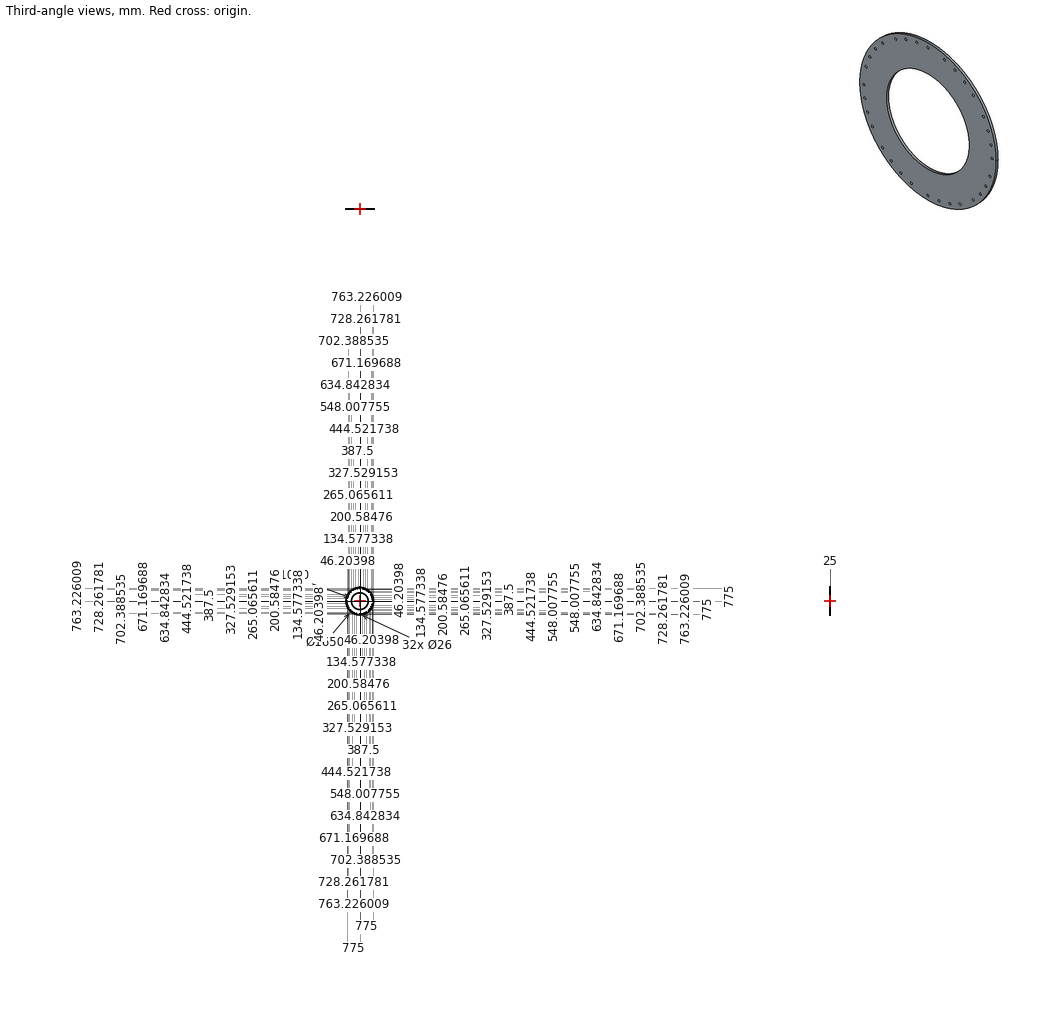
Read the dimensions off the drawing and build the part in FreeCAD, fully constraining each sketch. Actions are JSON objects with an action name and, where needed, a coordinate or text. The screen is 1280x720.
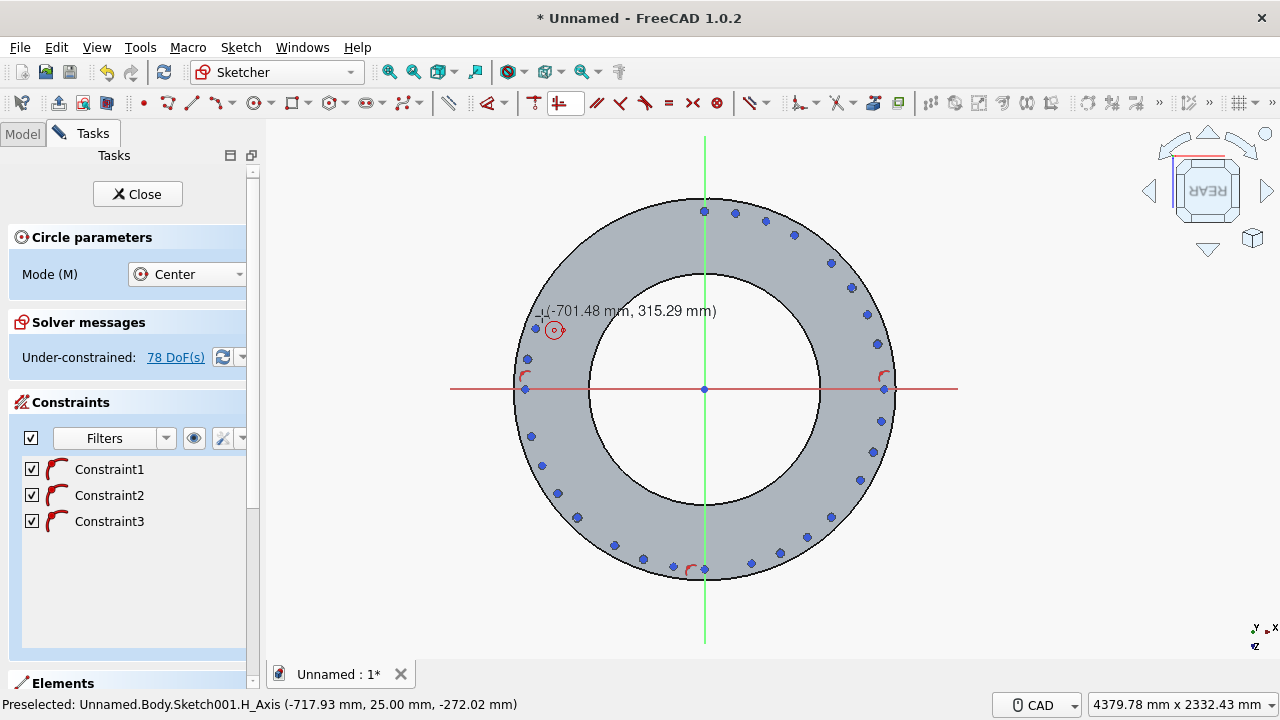
{"action": "left_click", "coordinate": [549, 300]}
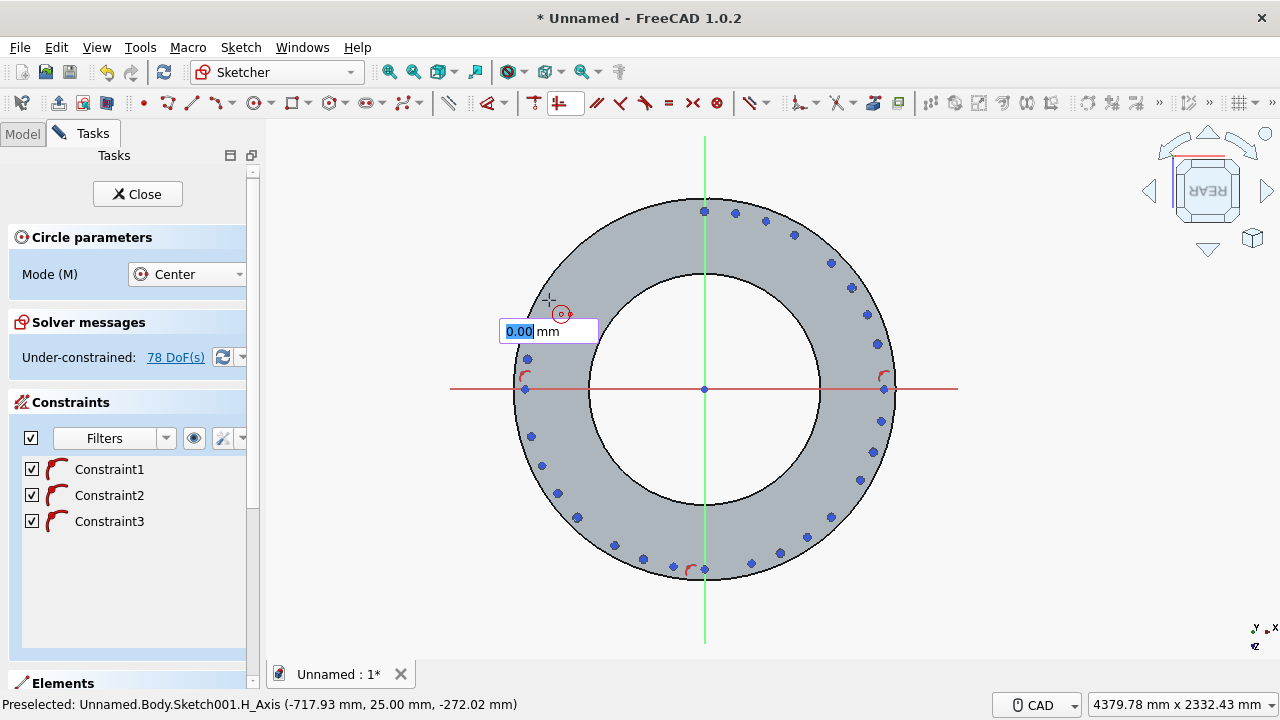
{"action": "scroll", "coordinate": [551, 298], "scroll_direction": "up", "scroll_amount": 9}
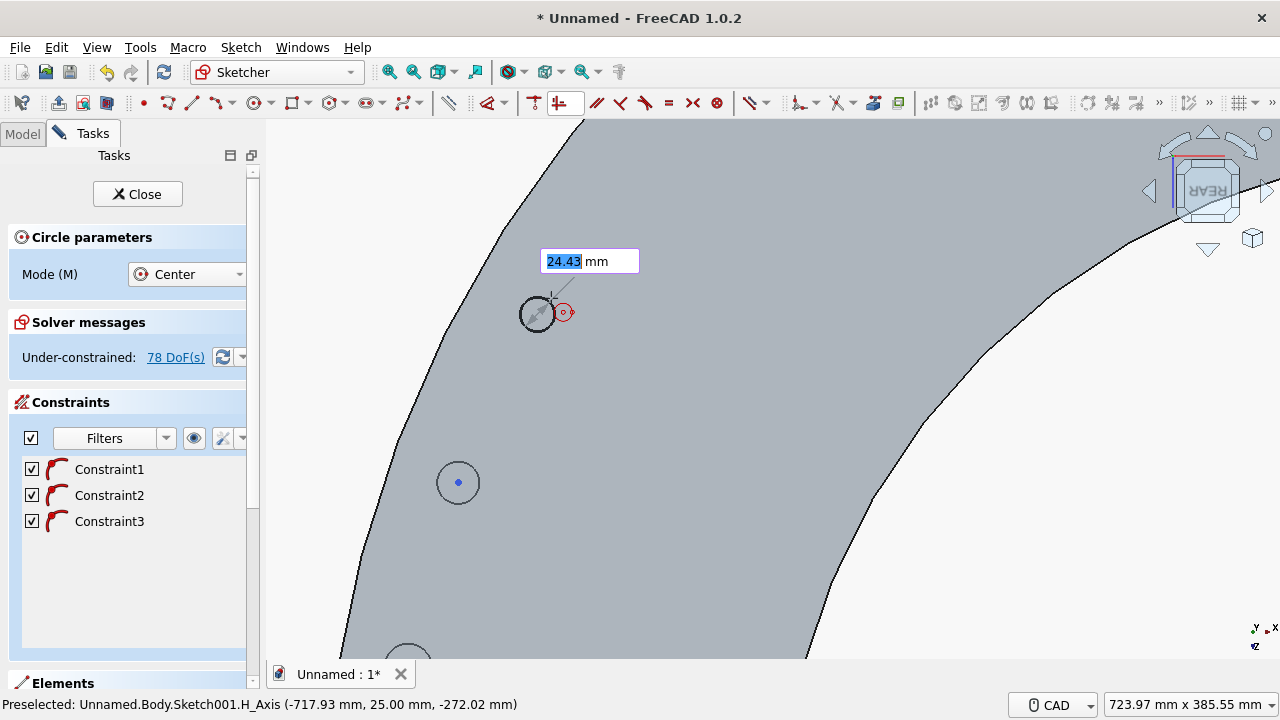
{"action": "left_click", "coordinate": [552, 294]}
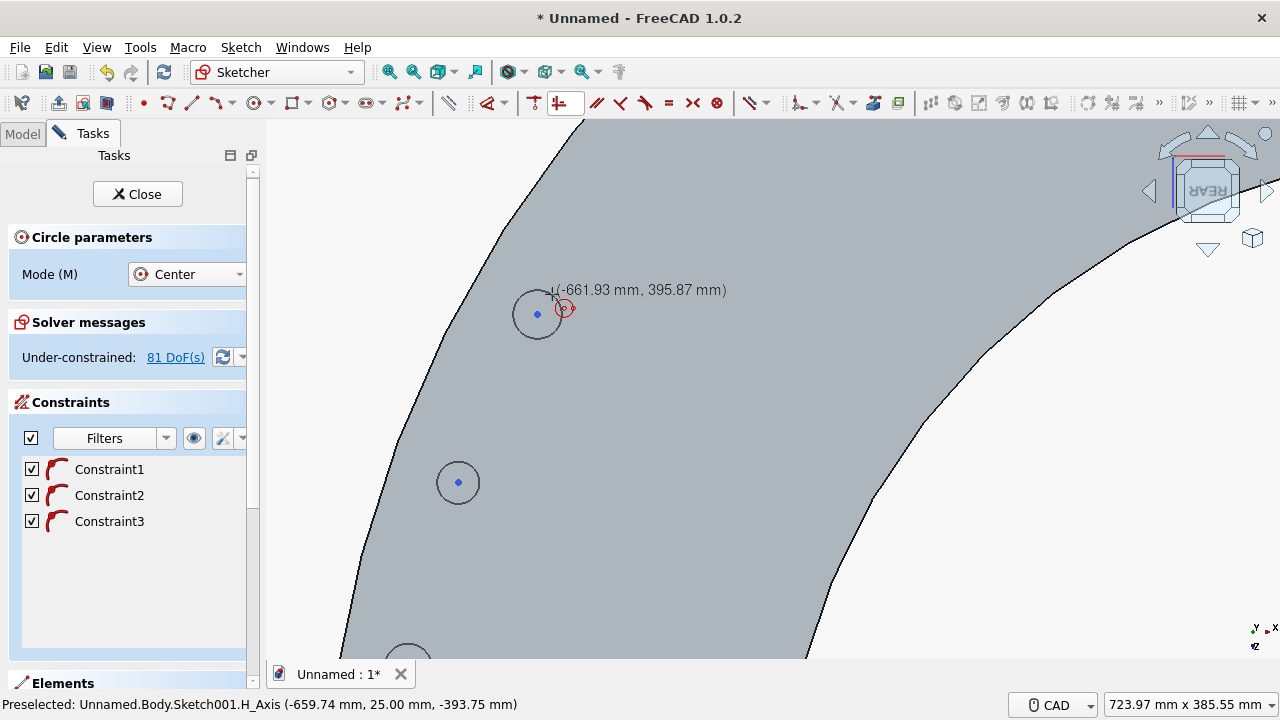
{"action": "scroll", "coordinate": [551, 298], "scroll_direction": "down", "scroll_amount": 9}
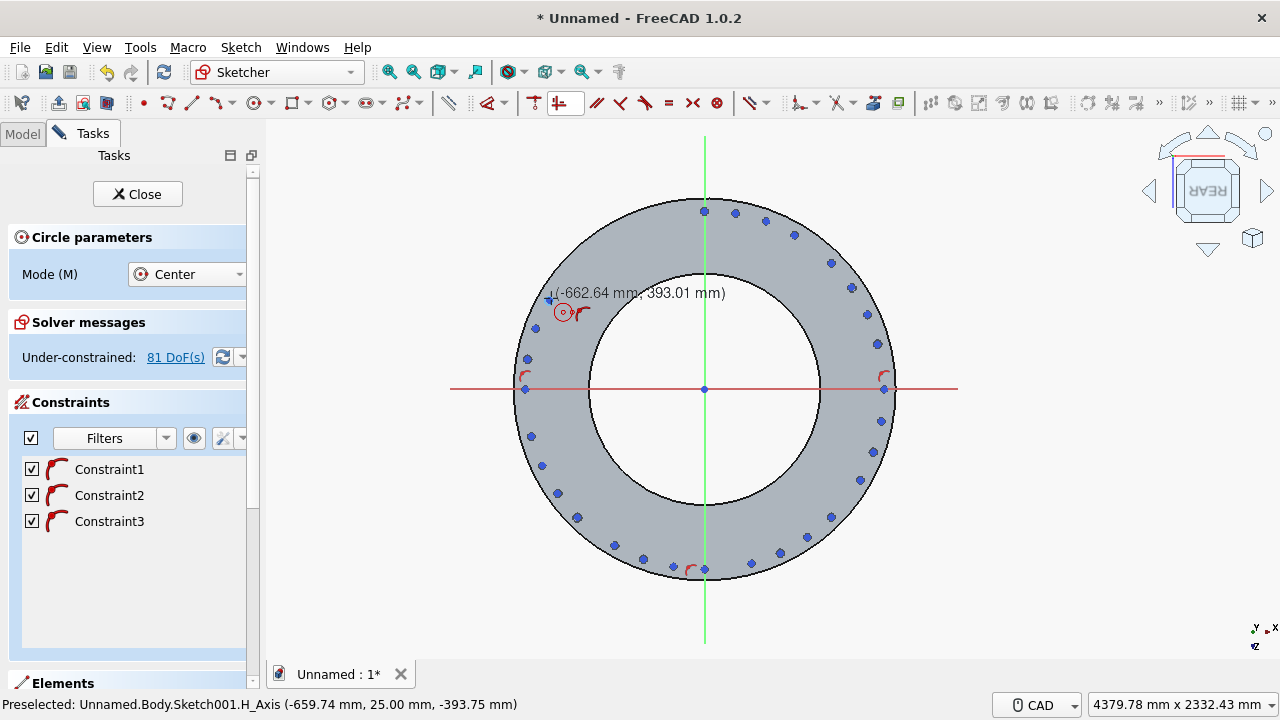
{"action": "scroll", "coordinate": [578, 263], "scroll_direction": "up", "scroll_amount": 11}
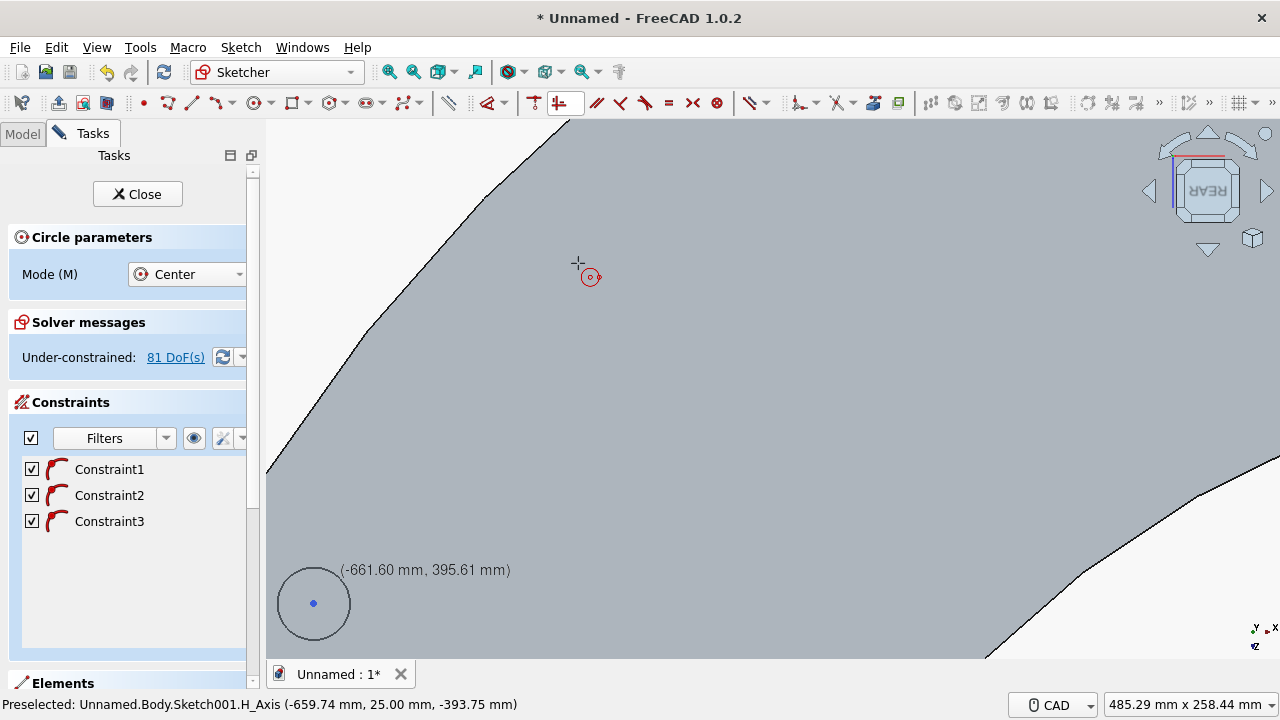
{"action": "scroll", "coordinate": [578, 263], "scroll_direction": "down", "scroll_amount": 11}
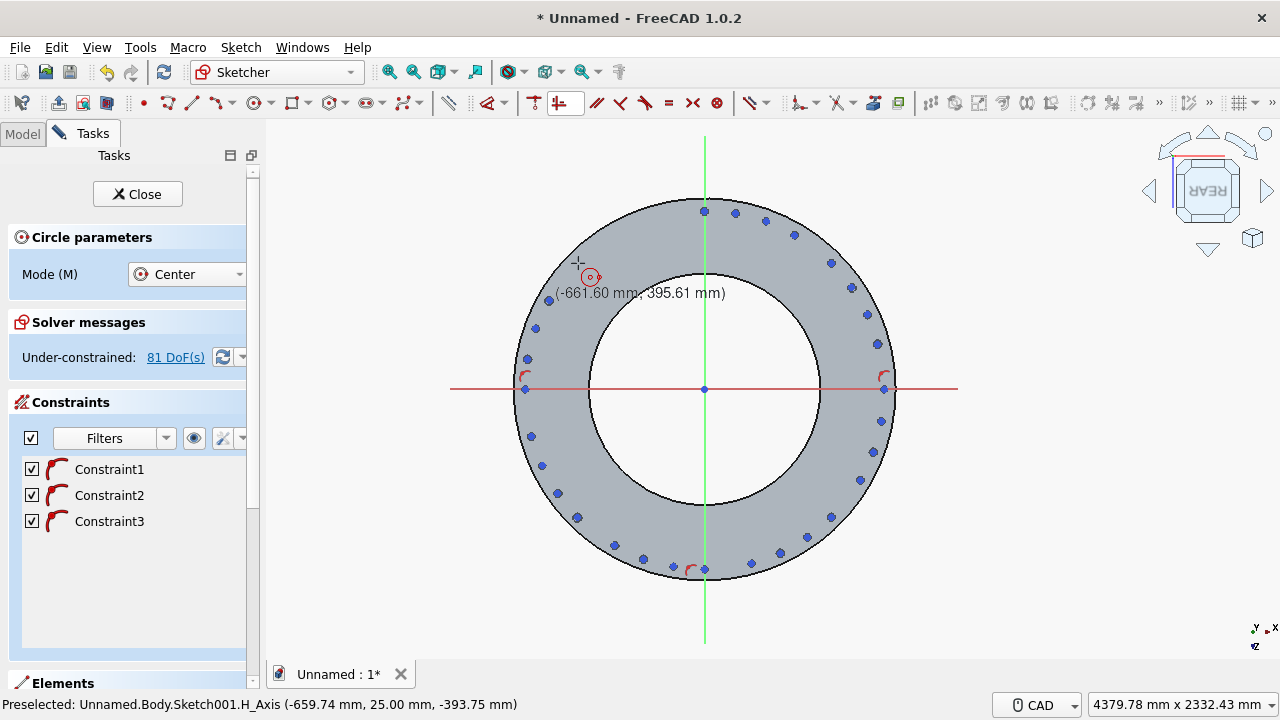
{"action": "left_click", "coordinate": [578, 263]}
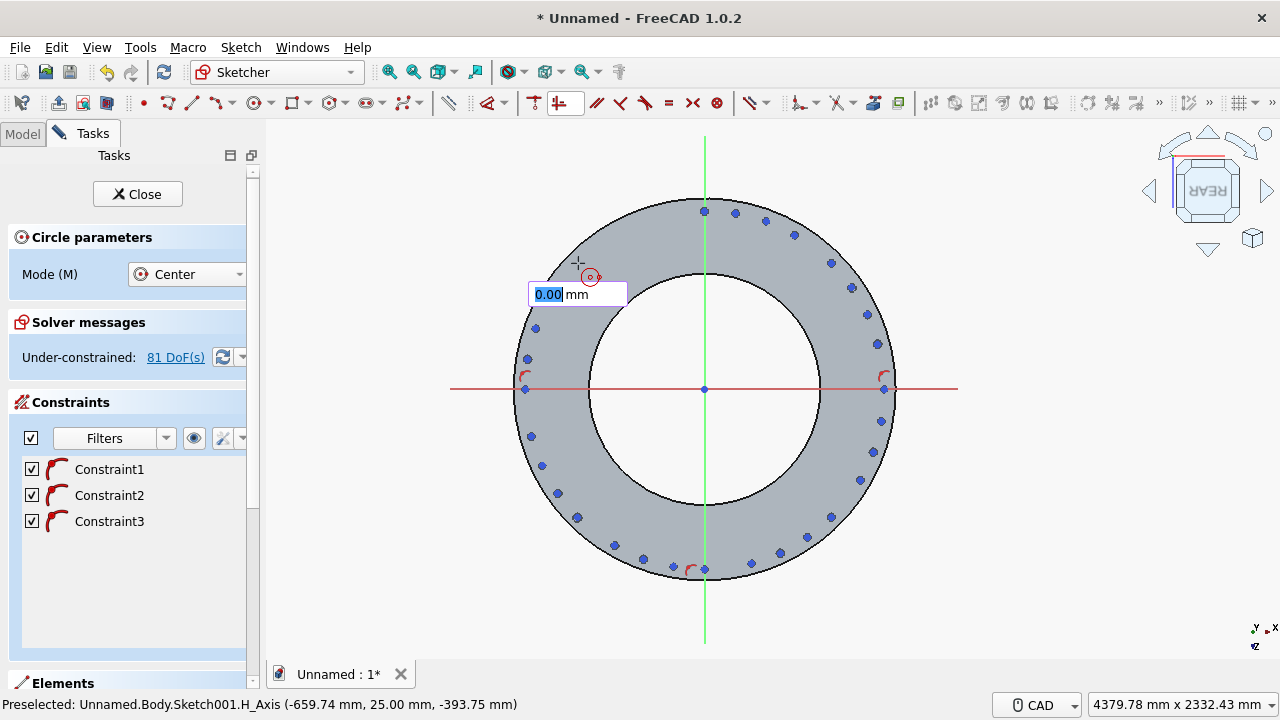
{"action": "scroll", "coordinate": [580, 260], "scroll_direction": "up", "scroll_amount": 9}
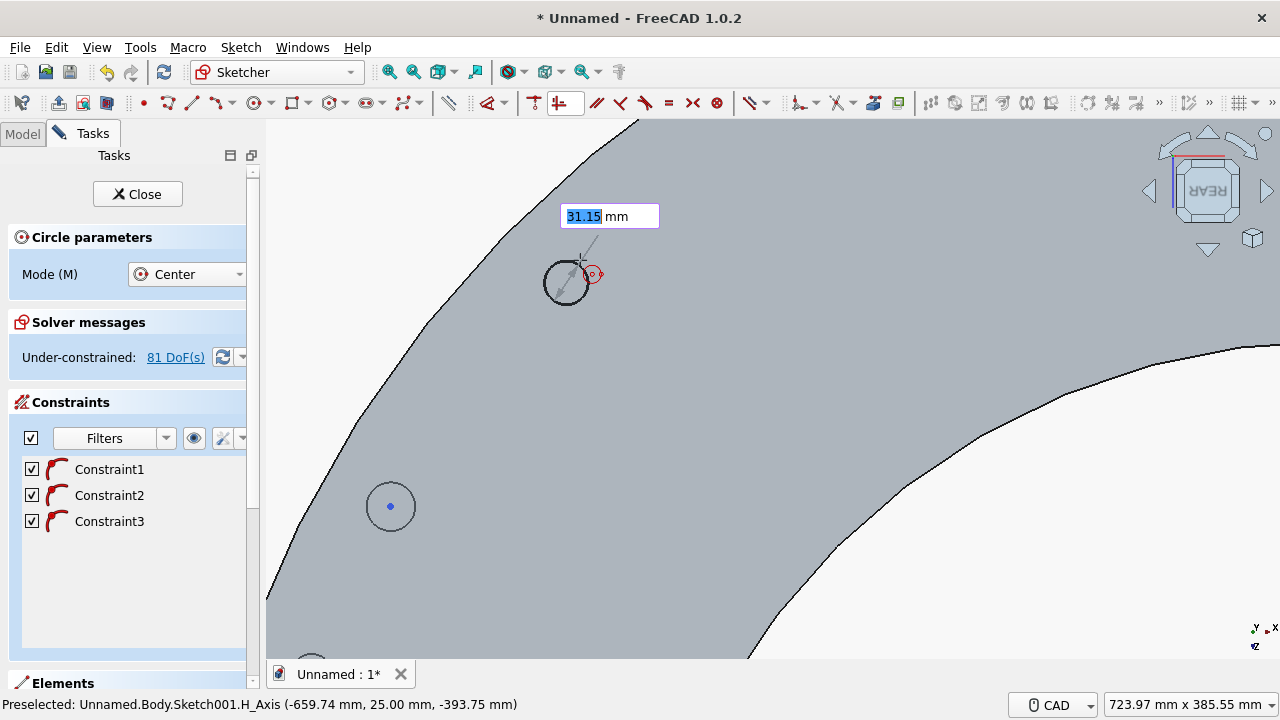
{"action": "left_click", "coordinate": [578, 261]}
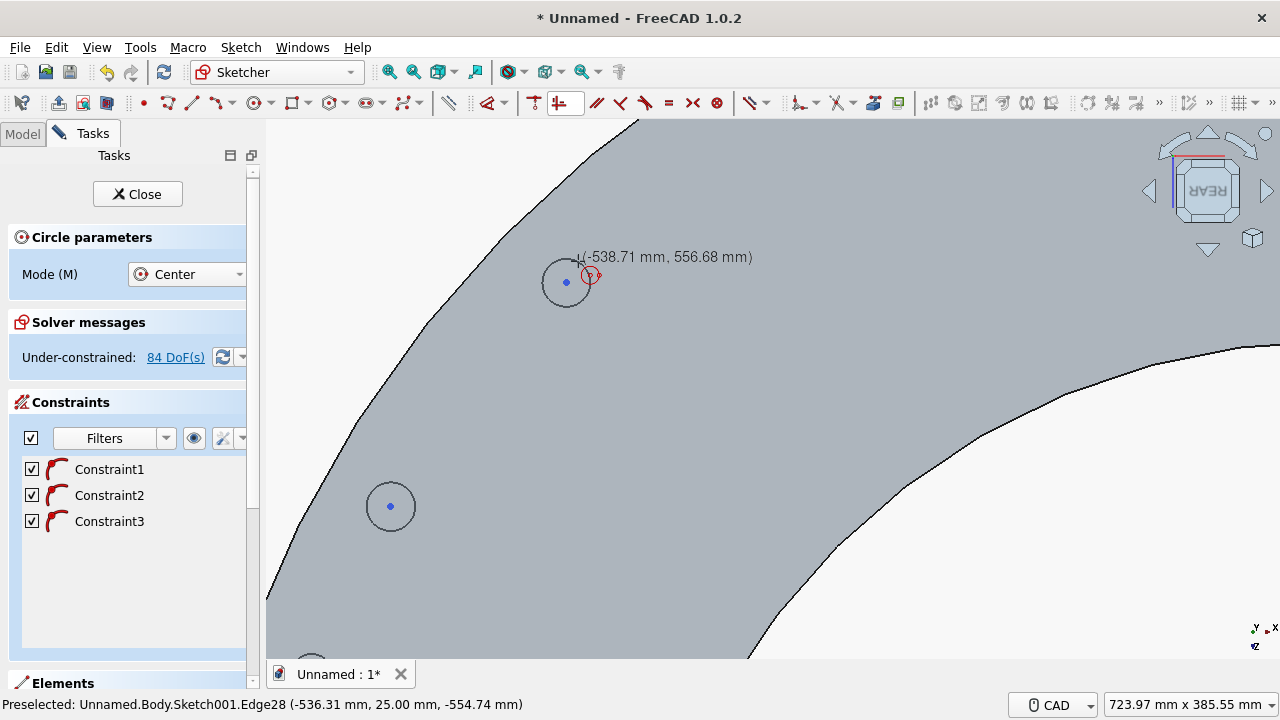
{"action": "scroll", "coordinate": [710, 153], "scroll_direction": "up", "scroll_amount": 2}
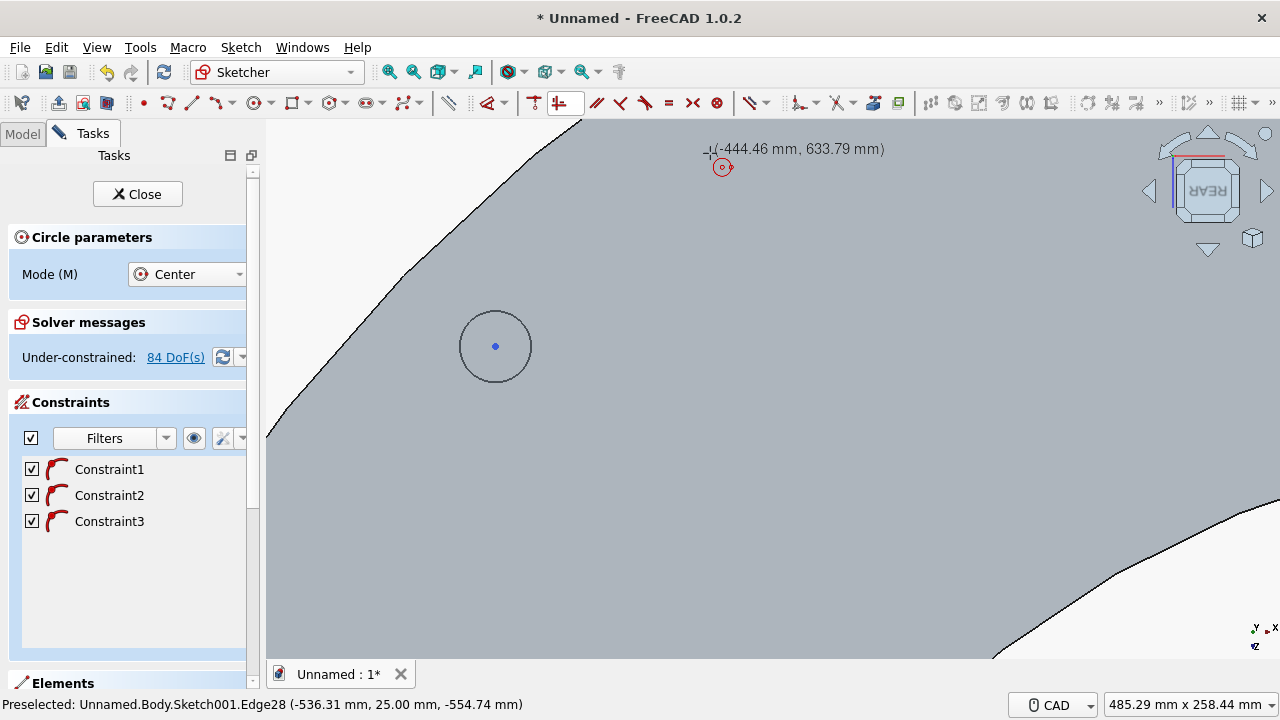
{"action": "scroll", "coordinate": [588, 253], "scroll_direction": "down", "scroll_amount": 11}